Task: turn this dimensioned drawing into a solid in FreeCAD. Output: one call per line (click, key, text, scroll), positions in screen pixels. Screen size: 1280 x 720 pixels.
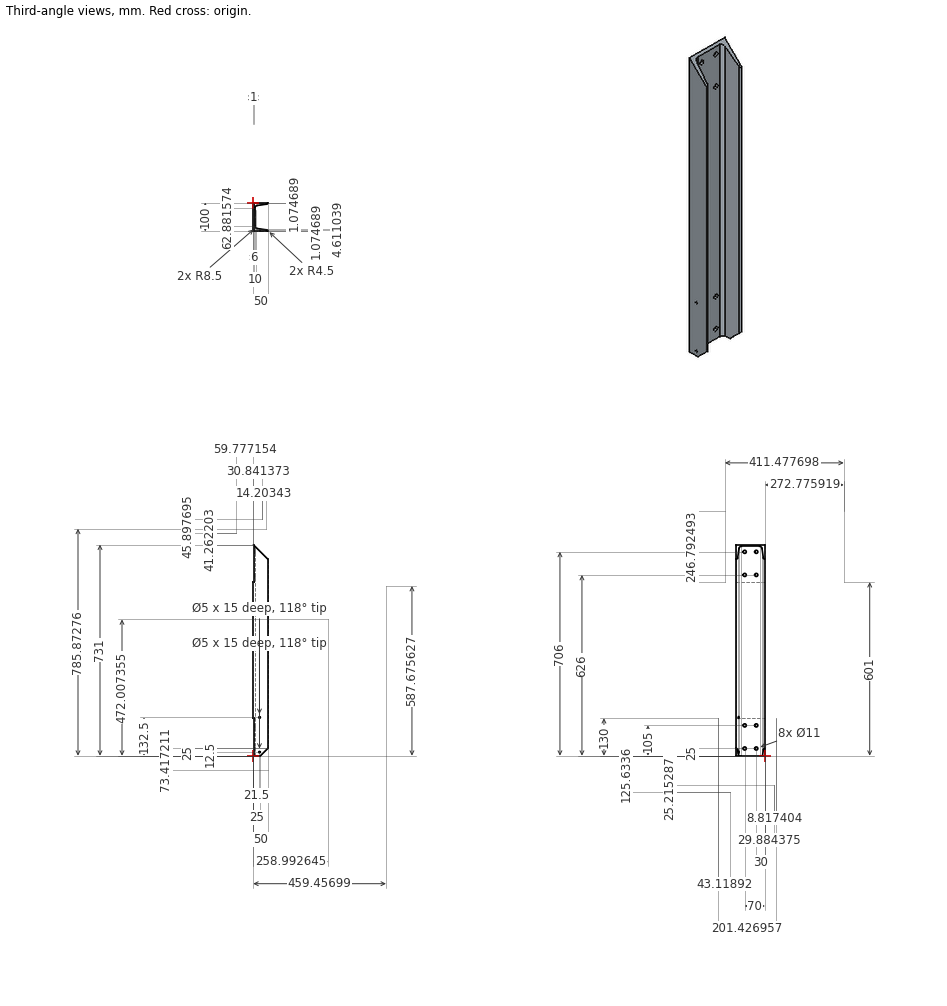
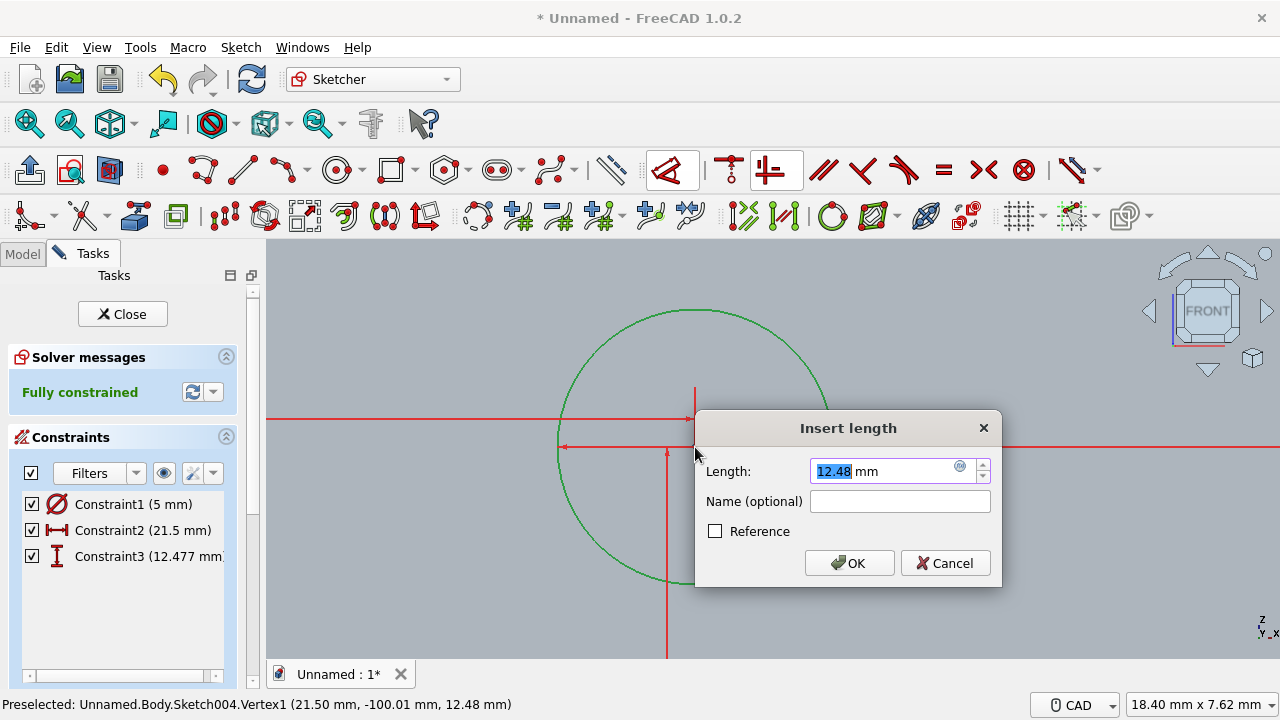
text(12.5)
key(Return)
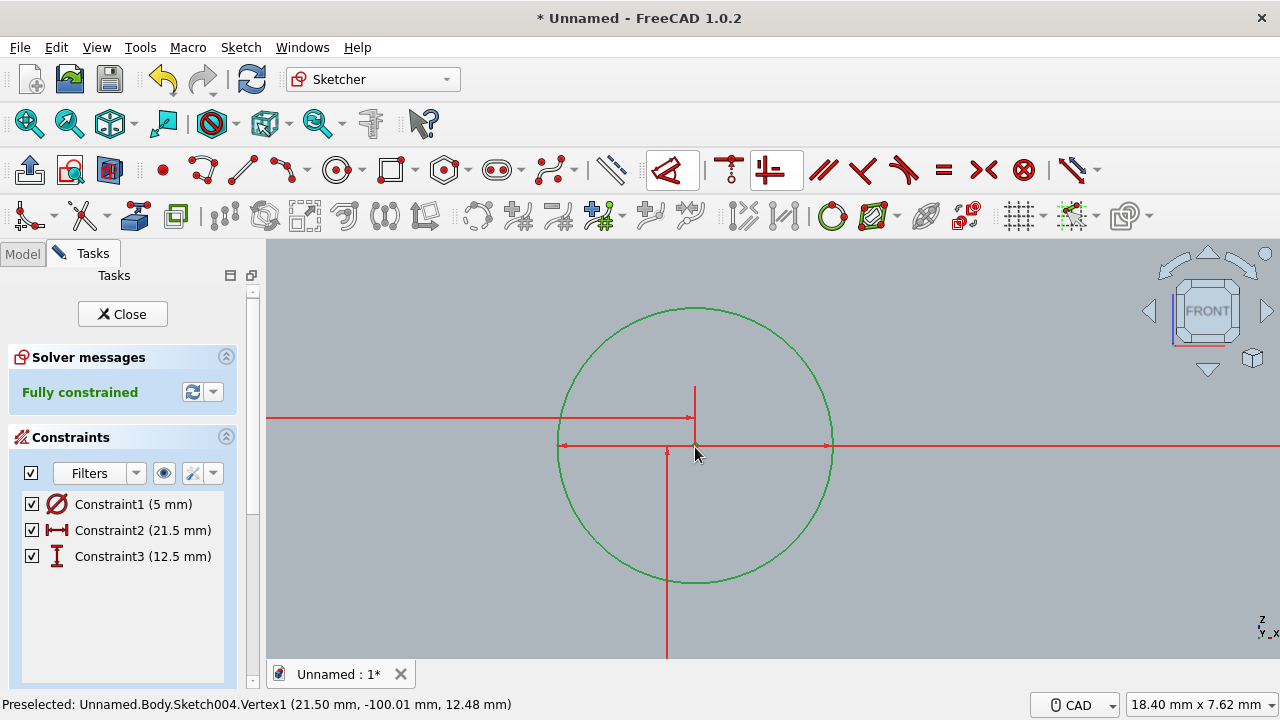
click(123, 314)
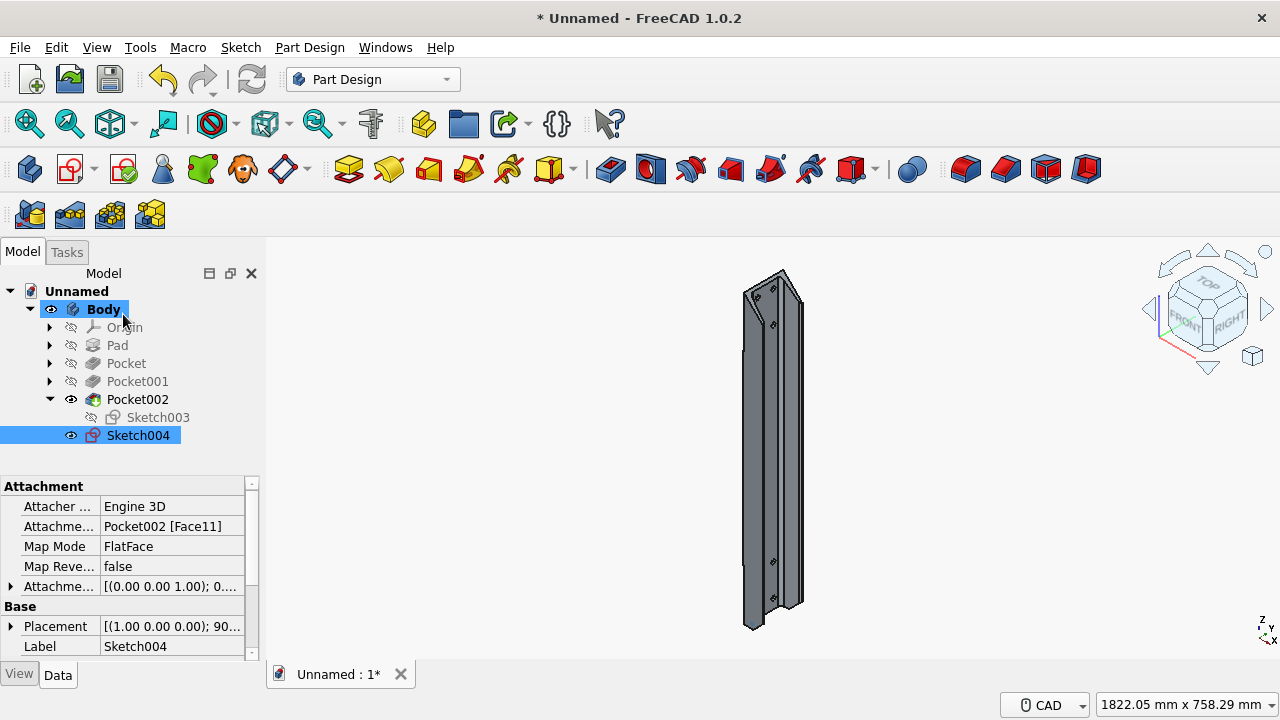
click(652, 170)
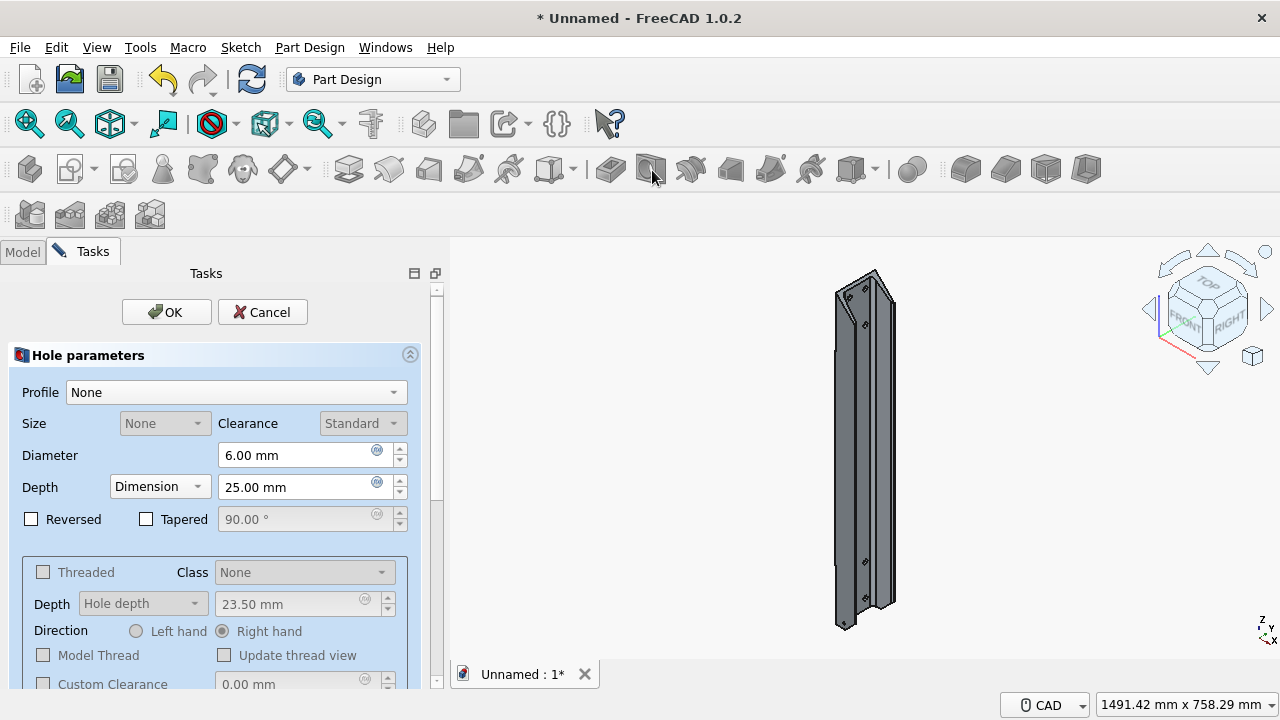
triple_click(305, 455)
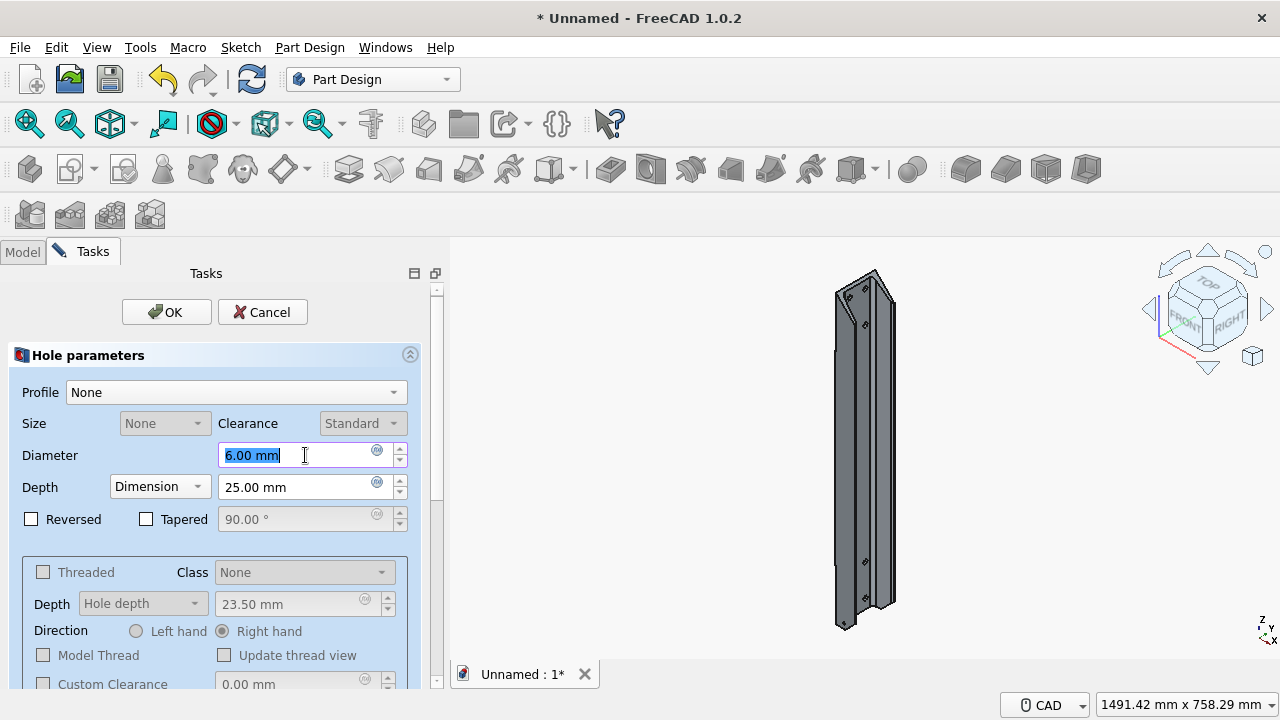
text(5)
key(Tab)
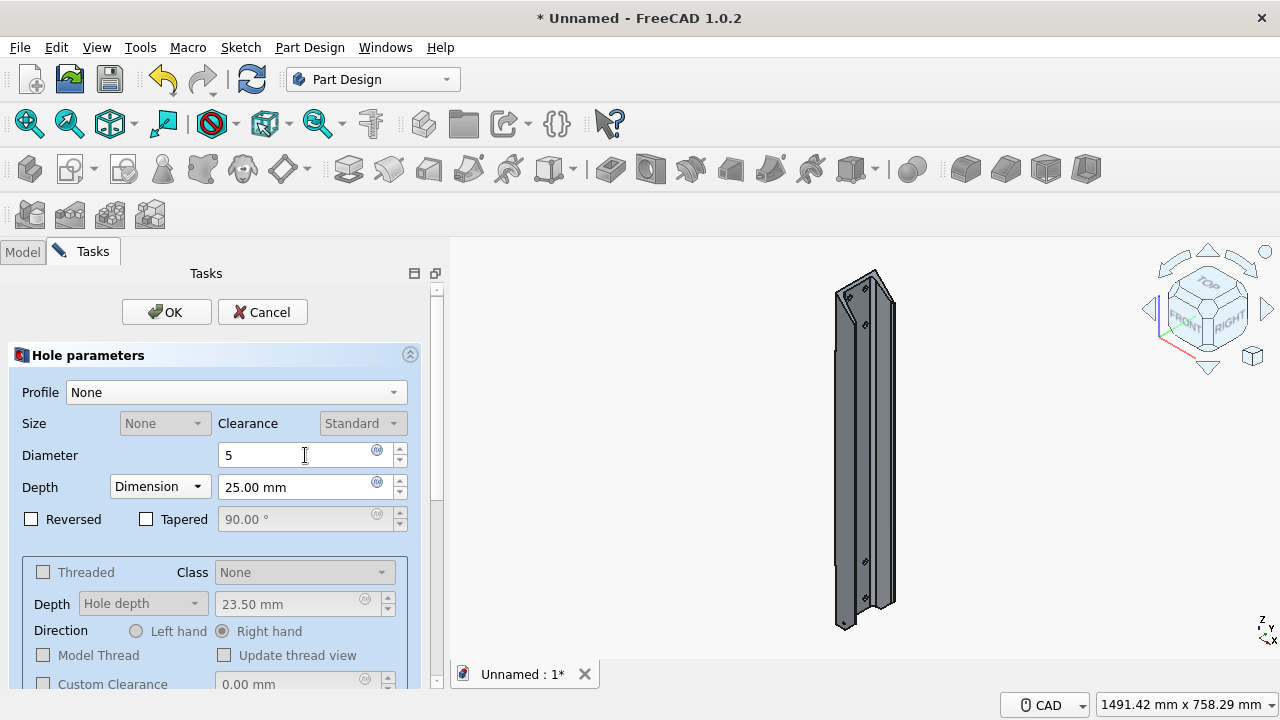
triple_click(305, 487)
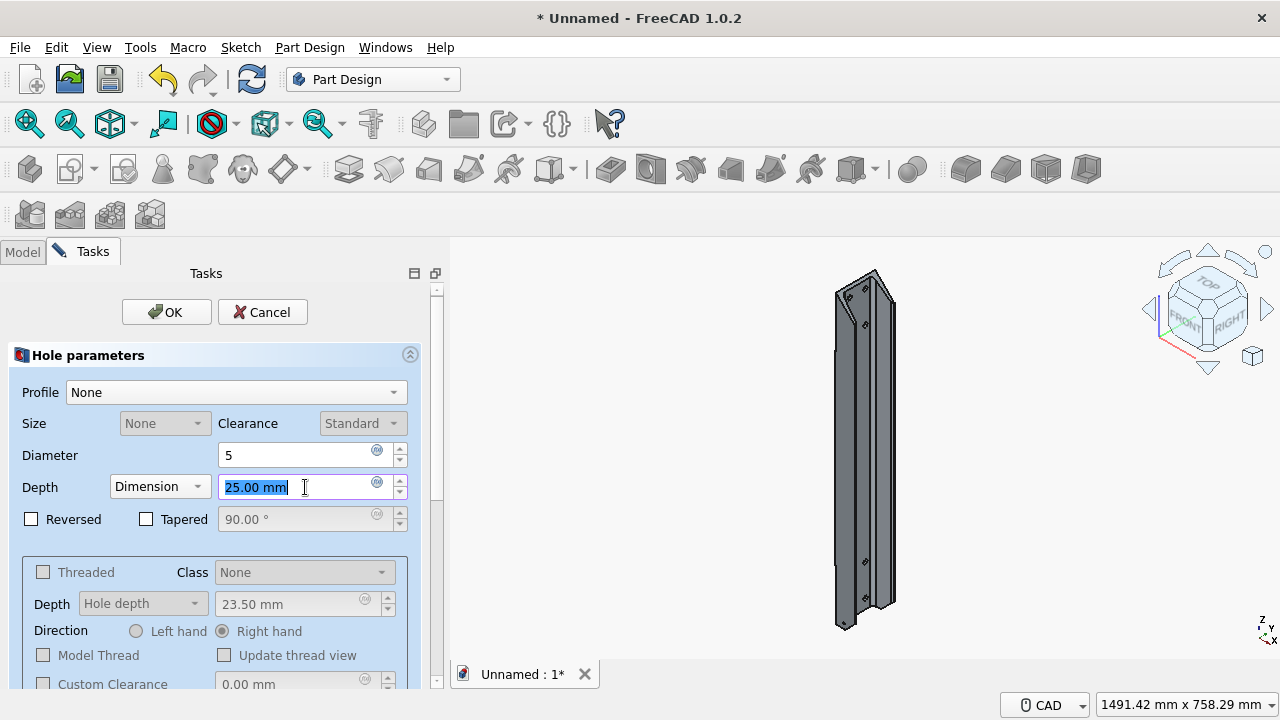
text(15)
key(Tab)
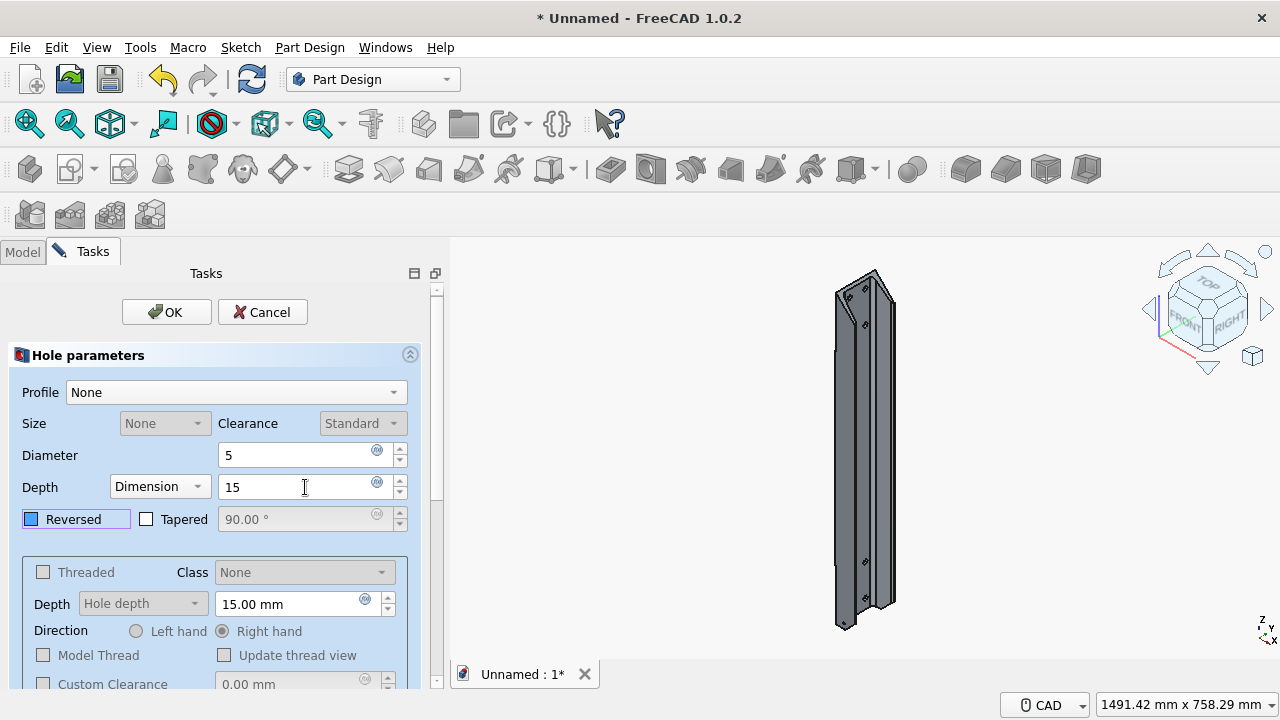
click(167, 312)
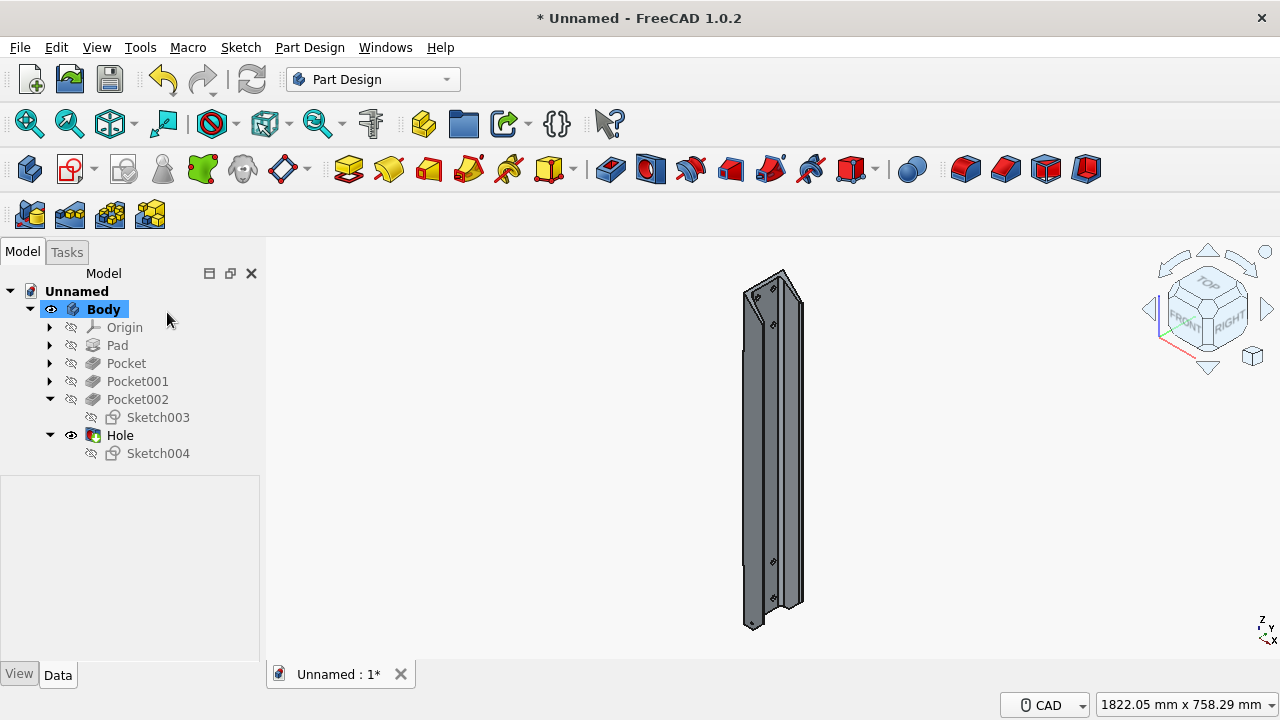
click(753, 368)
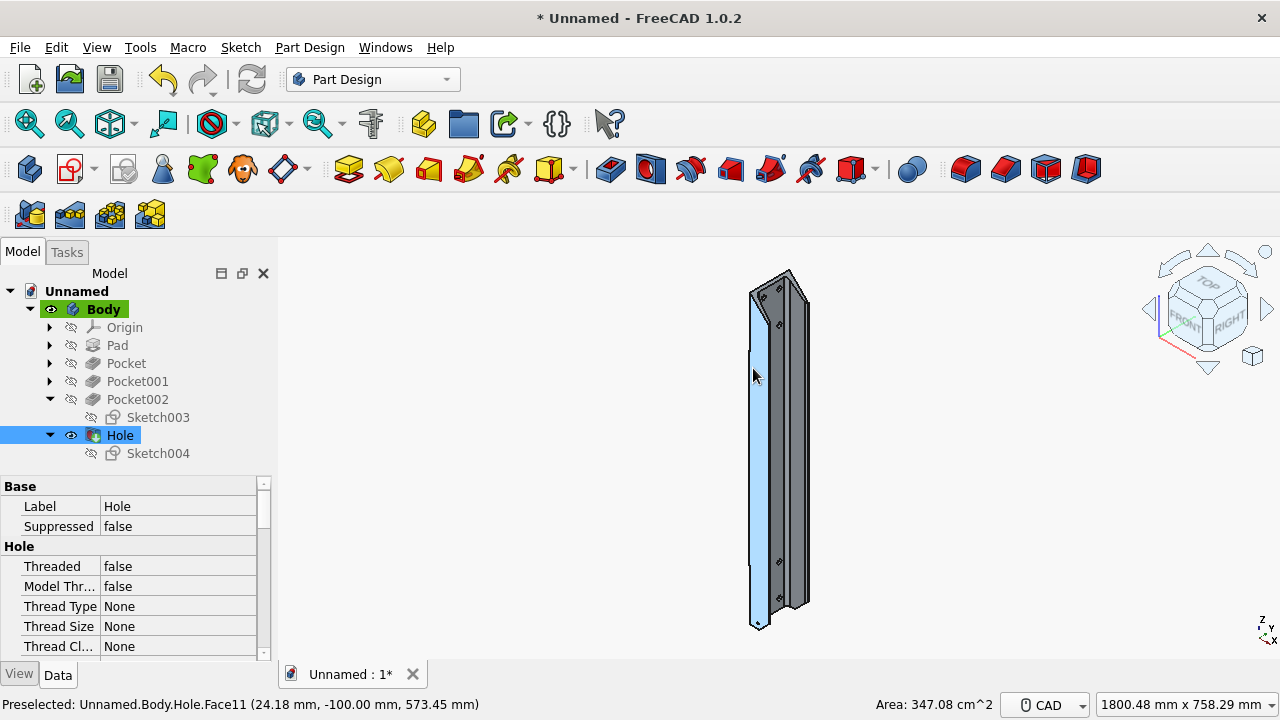
click(70, 170)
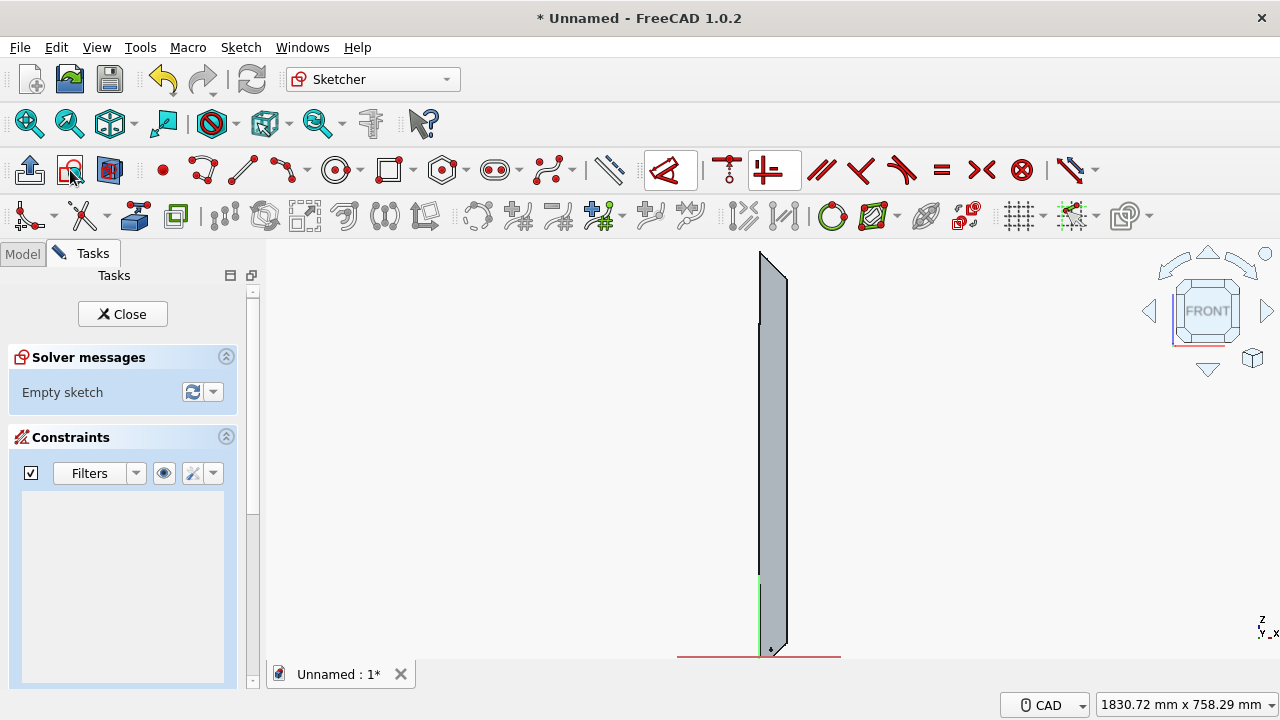
scroll(775, 590, up, 15)